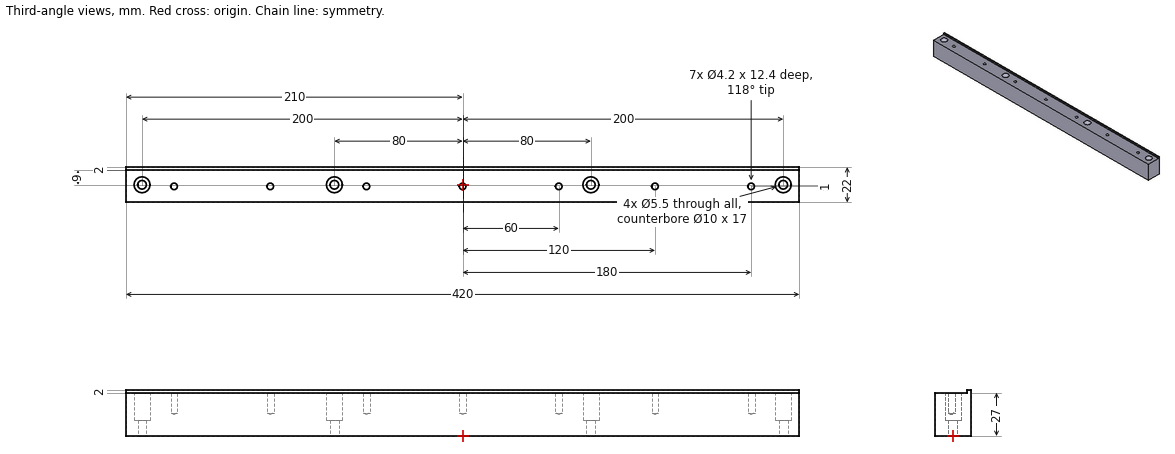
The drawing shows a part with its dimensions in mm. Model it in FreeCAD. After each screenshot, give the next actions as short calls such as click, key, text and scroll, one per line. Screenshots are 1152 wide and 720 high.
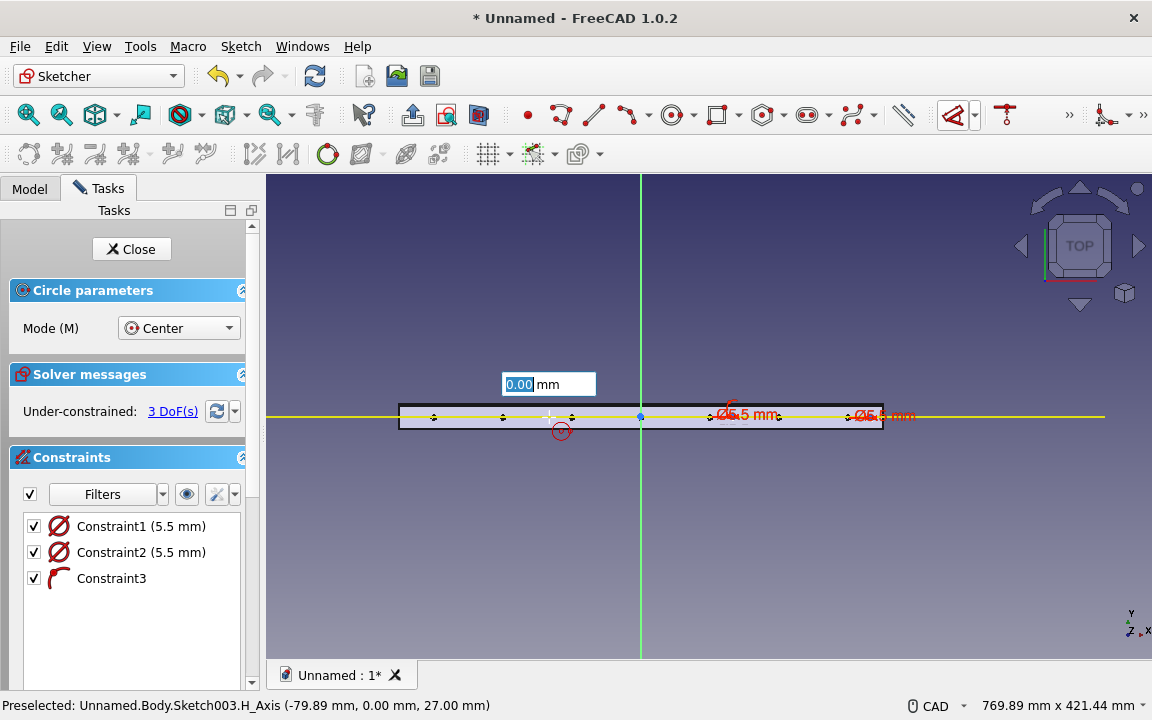
scroll(550, 414, up, 9)
move(548, 410)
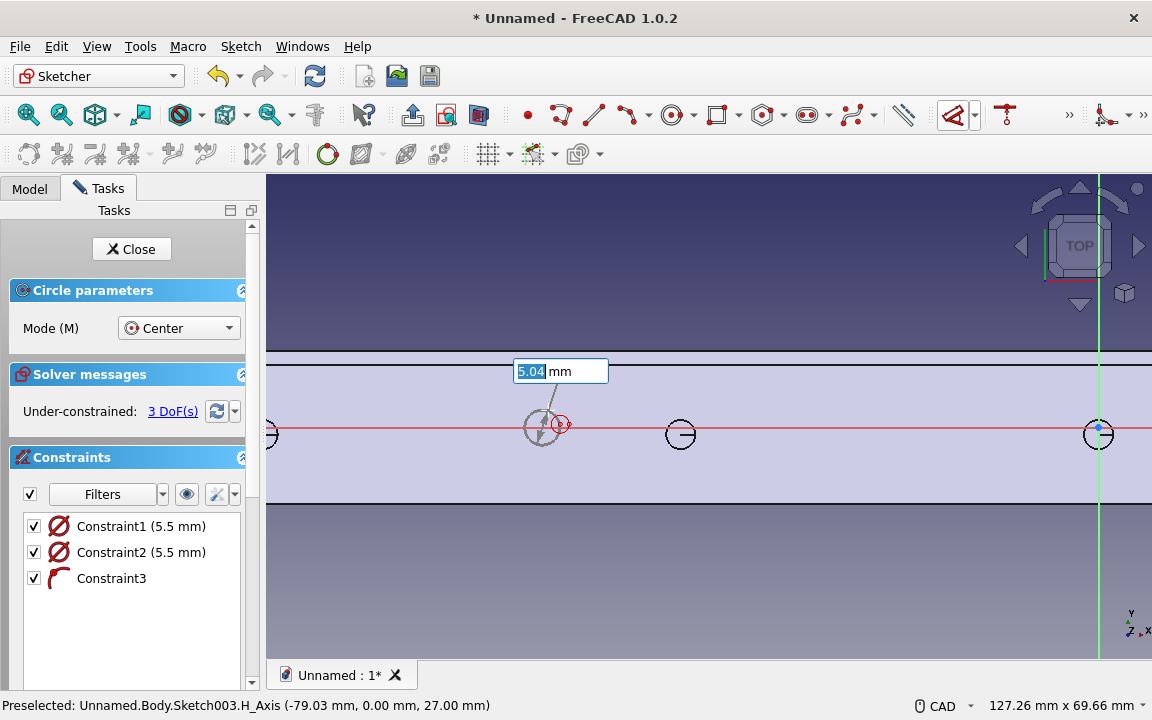
text(5.5)
key(Return)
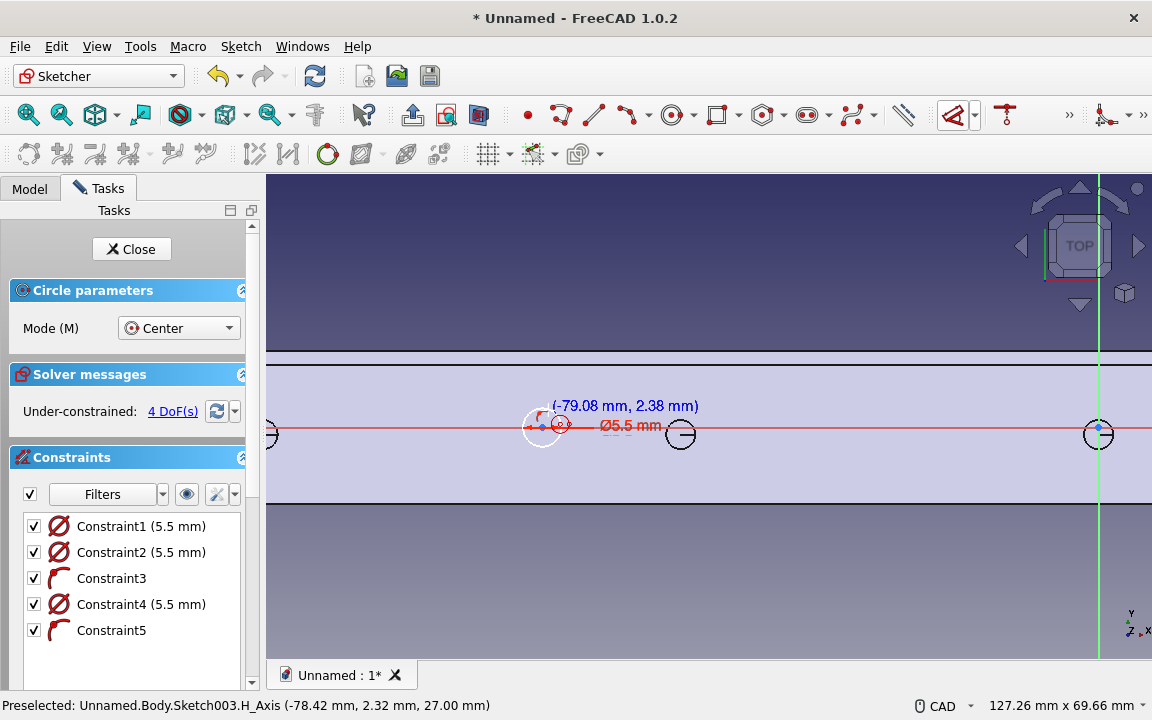
scroll(550, 414, down, 9)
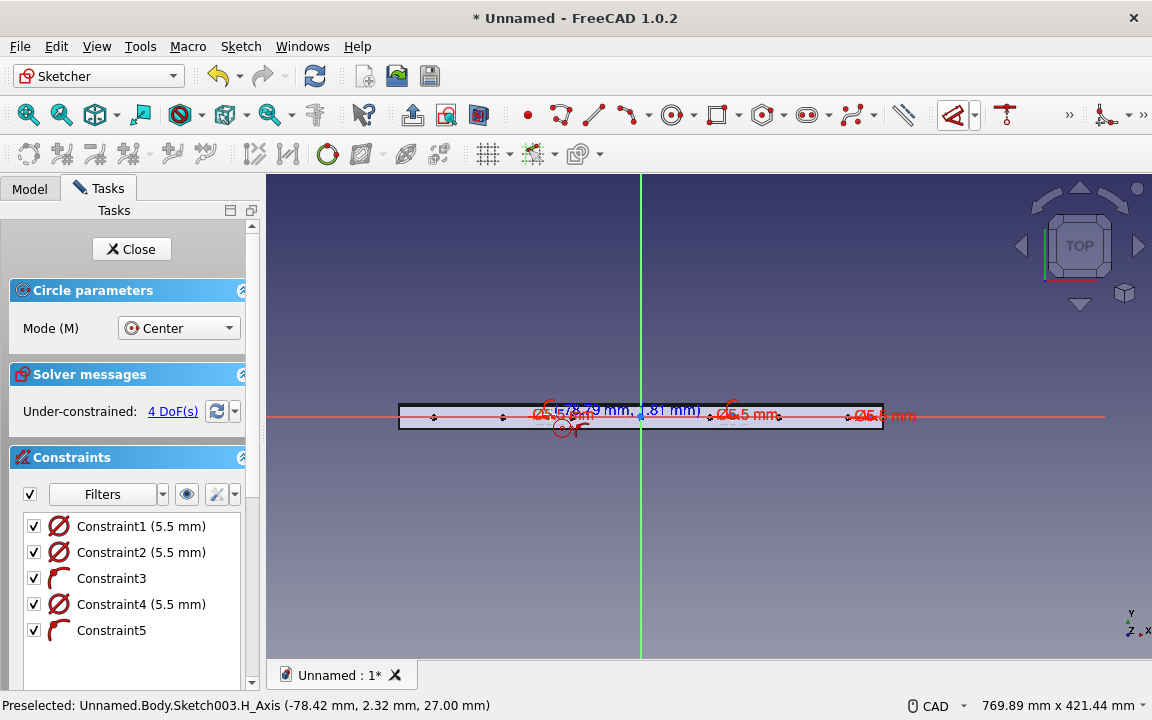
scroll(411, 417, up, 10)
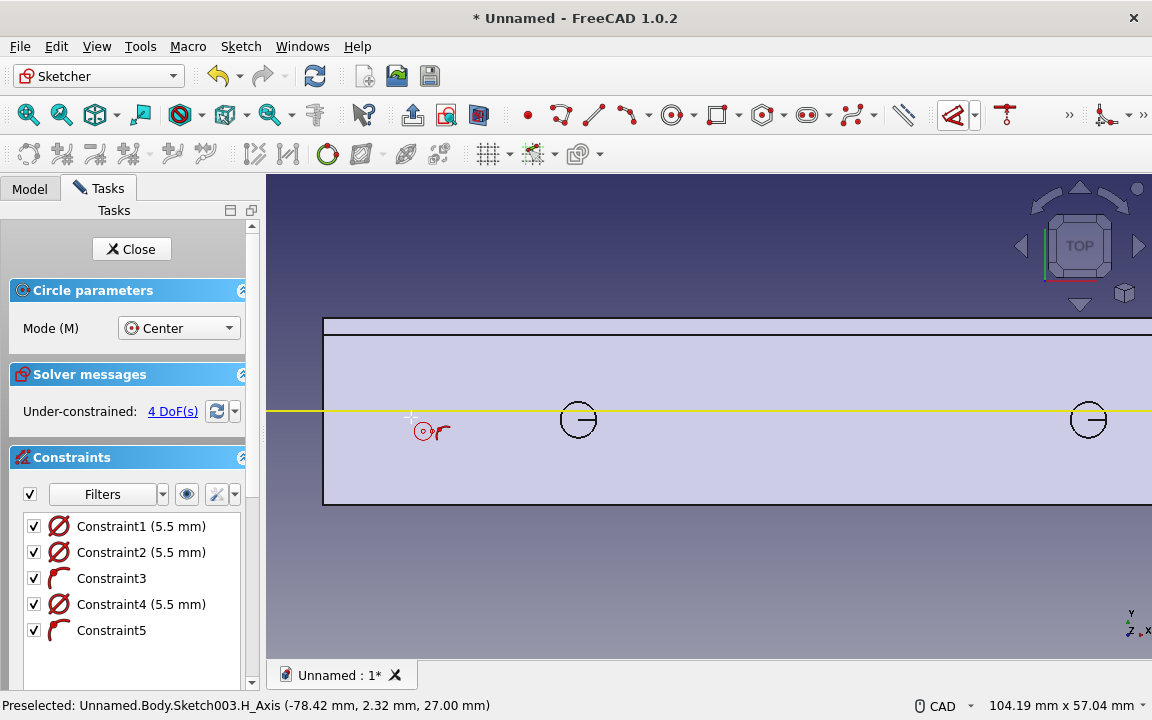
scroll(411, 417, down, 10)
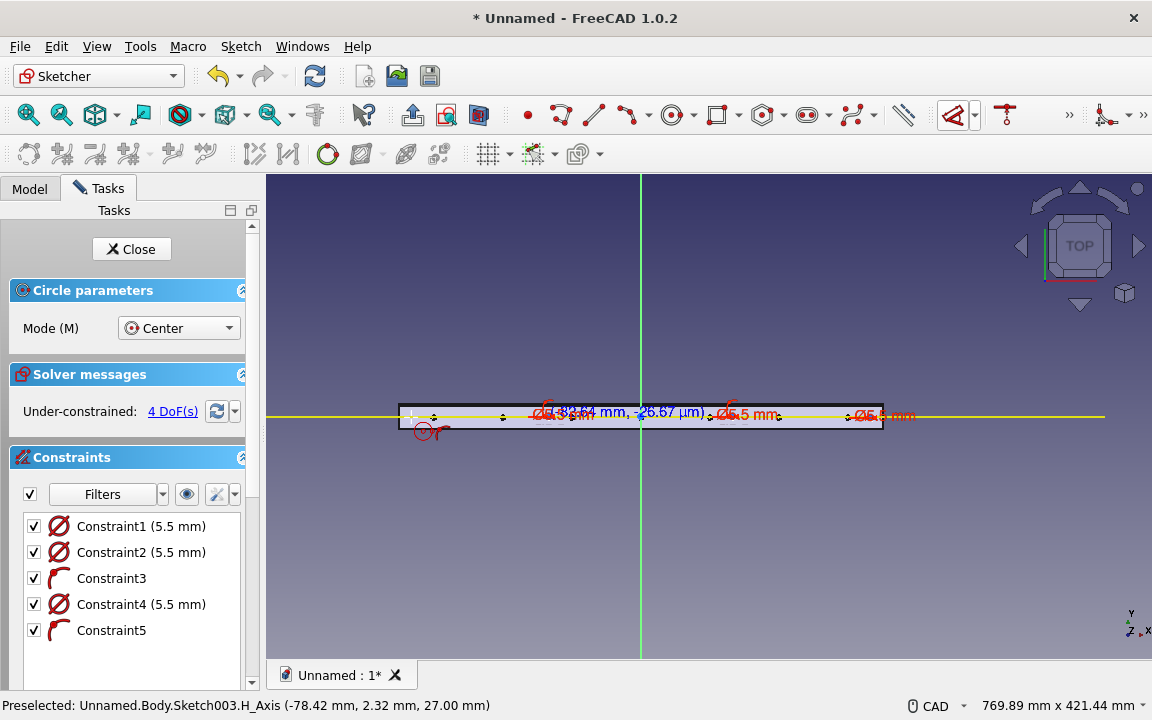
click(411, 417)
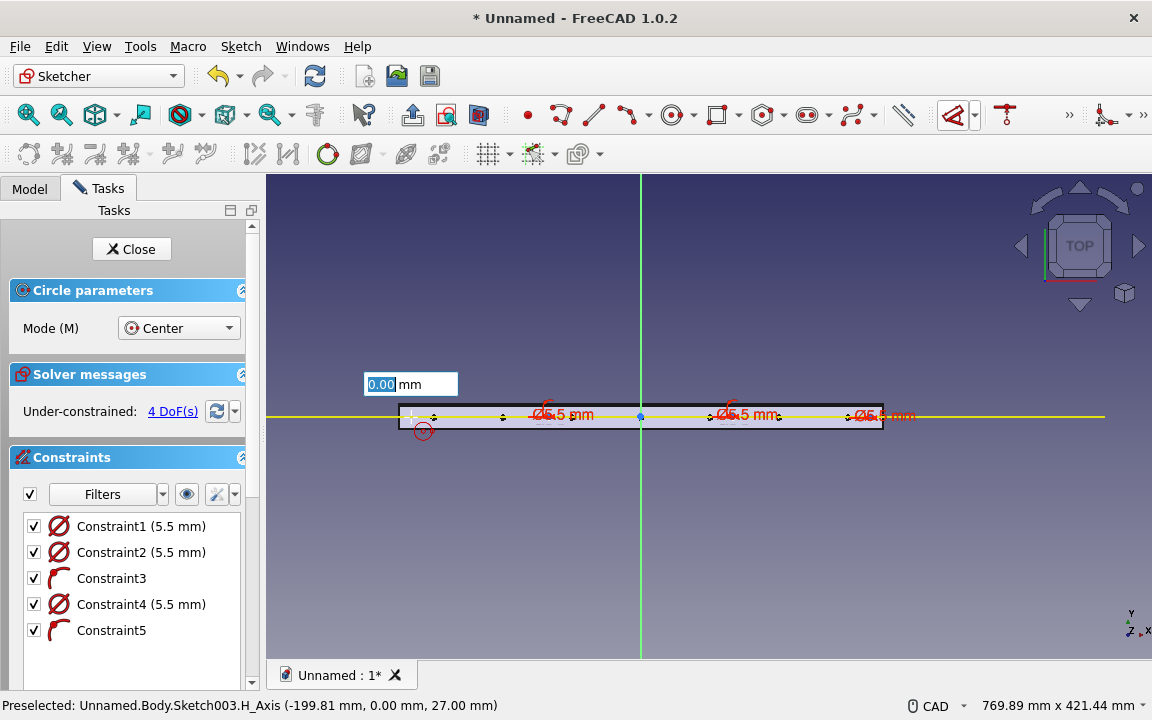
scroll(412, 414, up, 9)
move(410, 410)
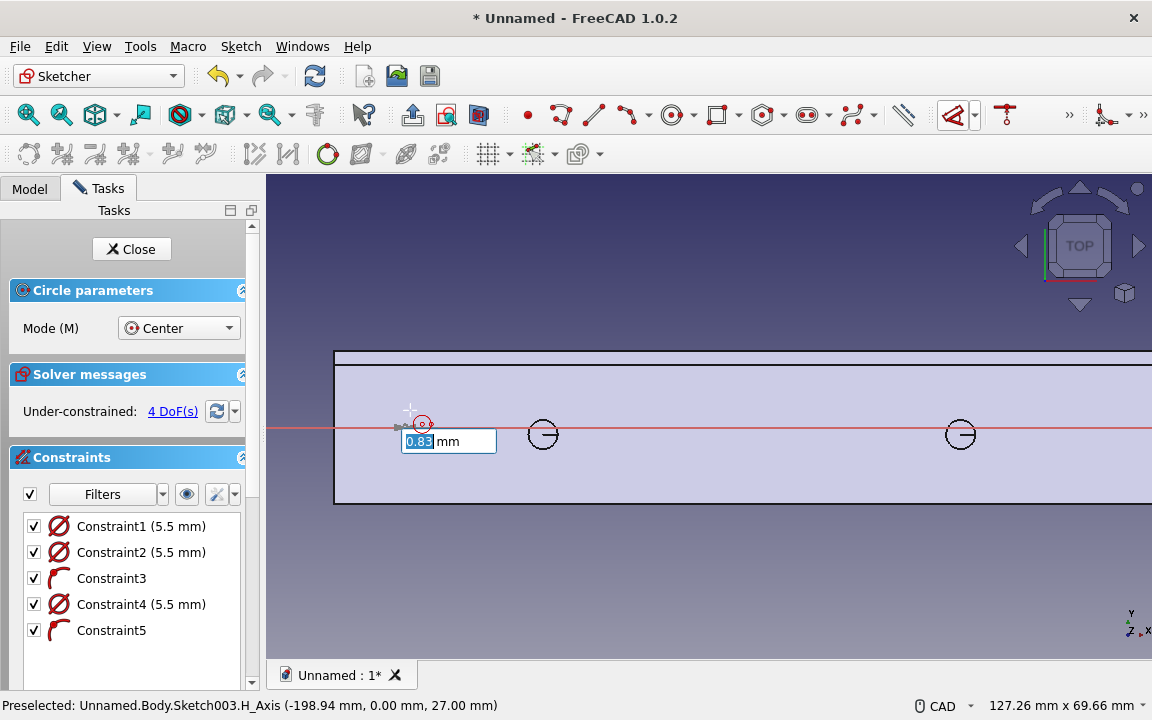
text(5.5)
key(Return)
key(Escape)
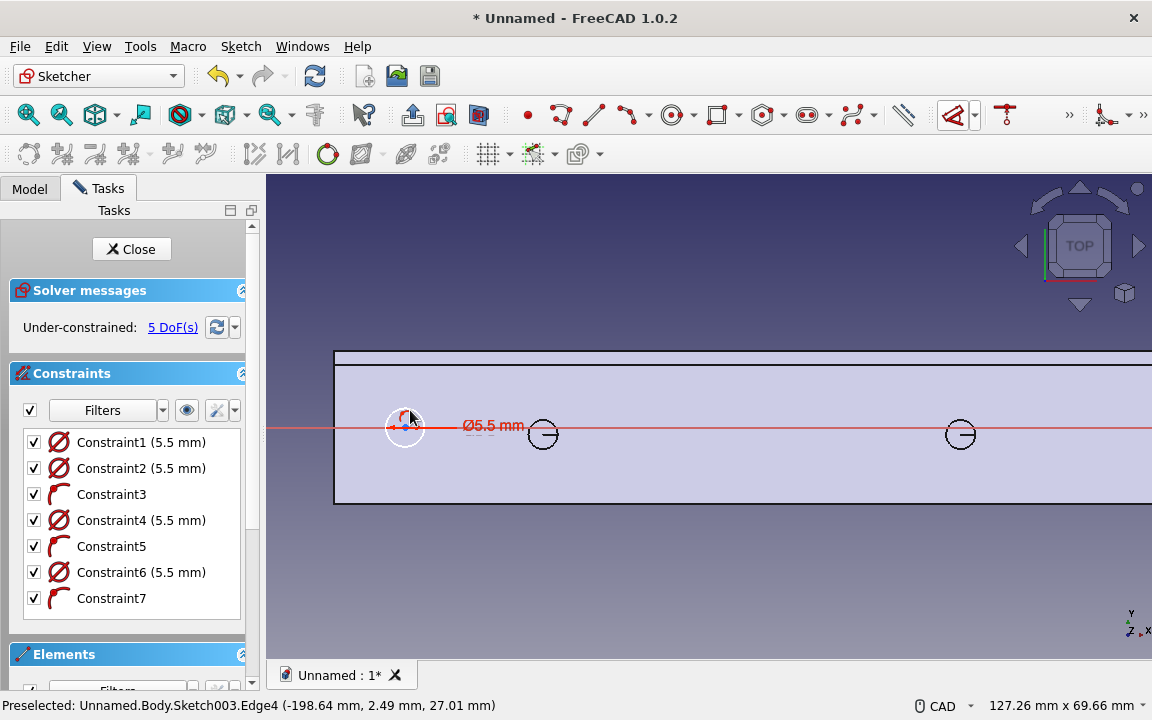
scroll(412, 414, down, 9)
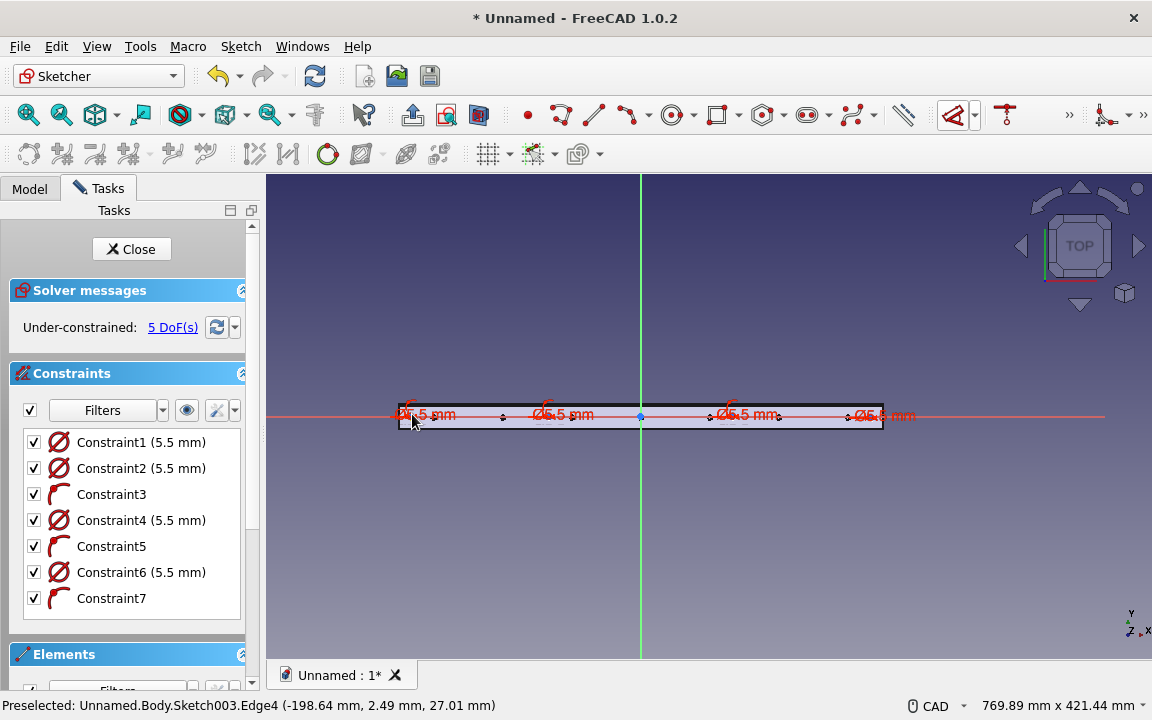
click(871, 418)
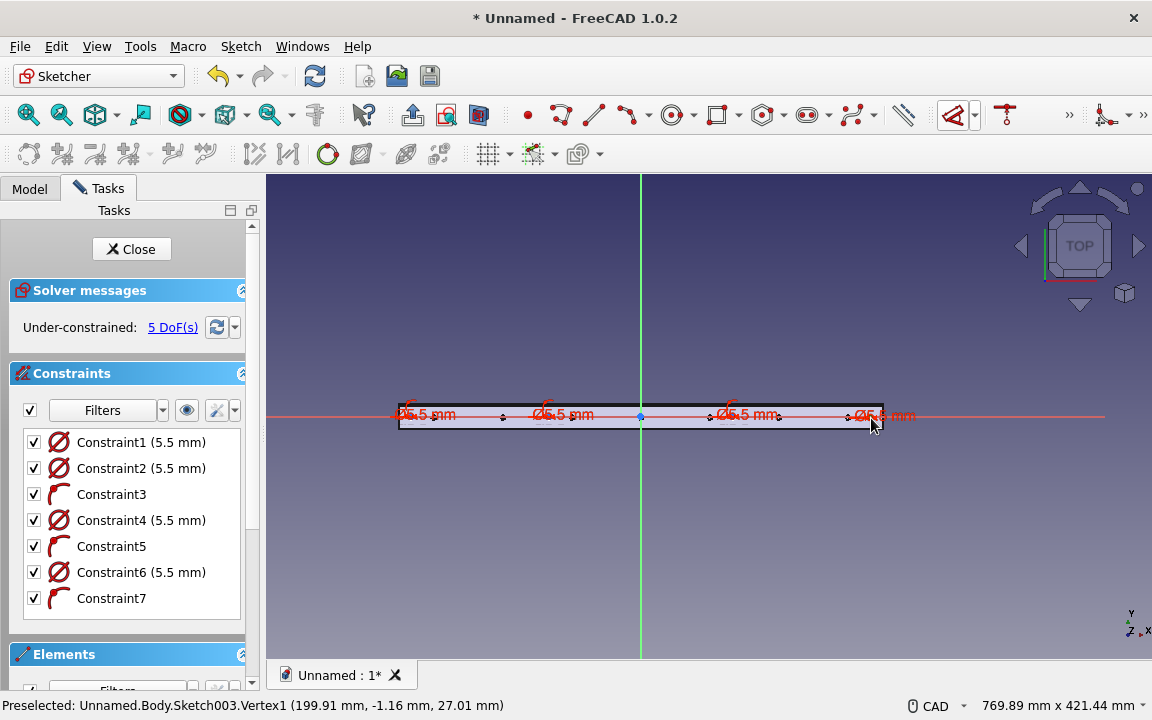
click(343, 417)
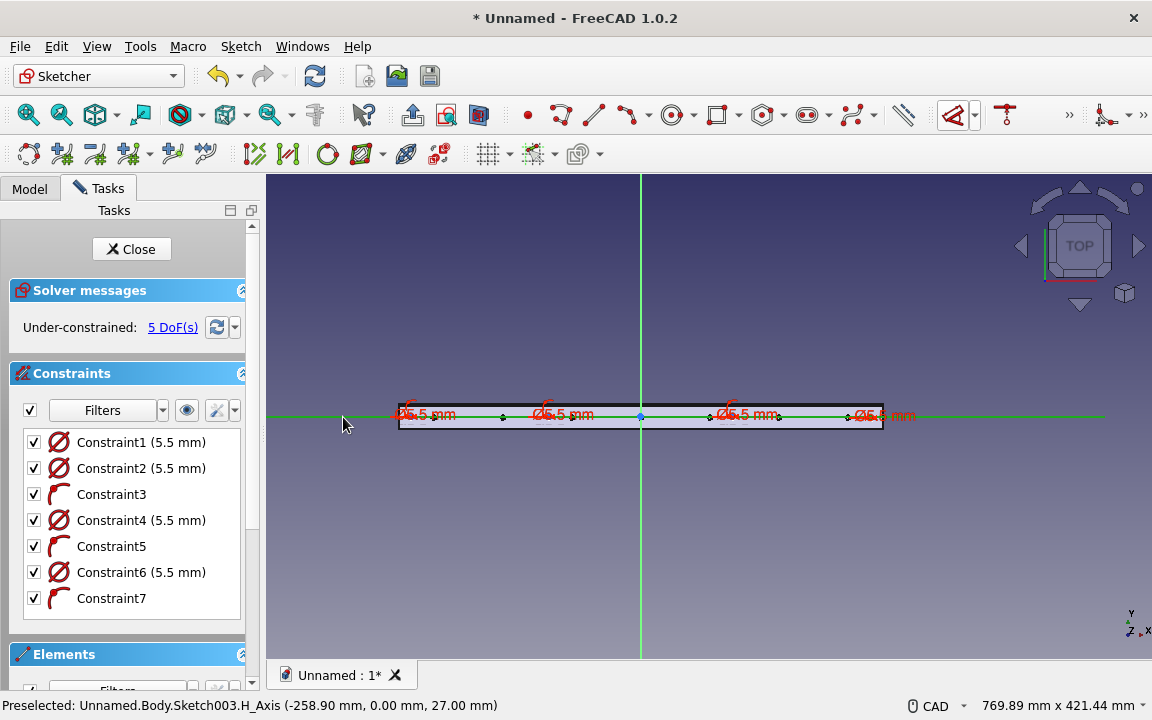
click(1005, 116)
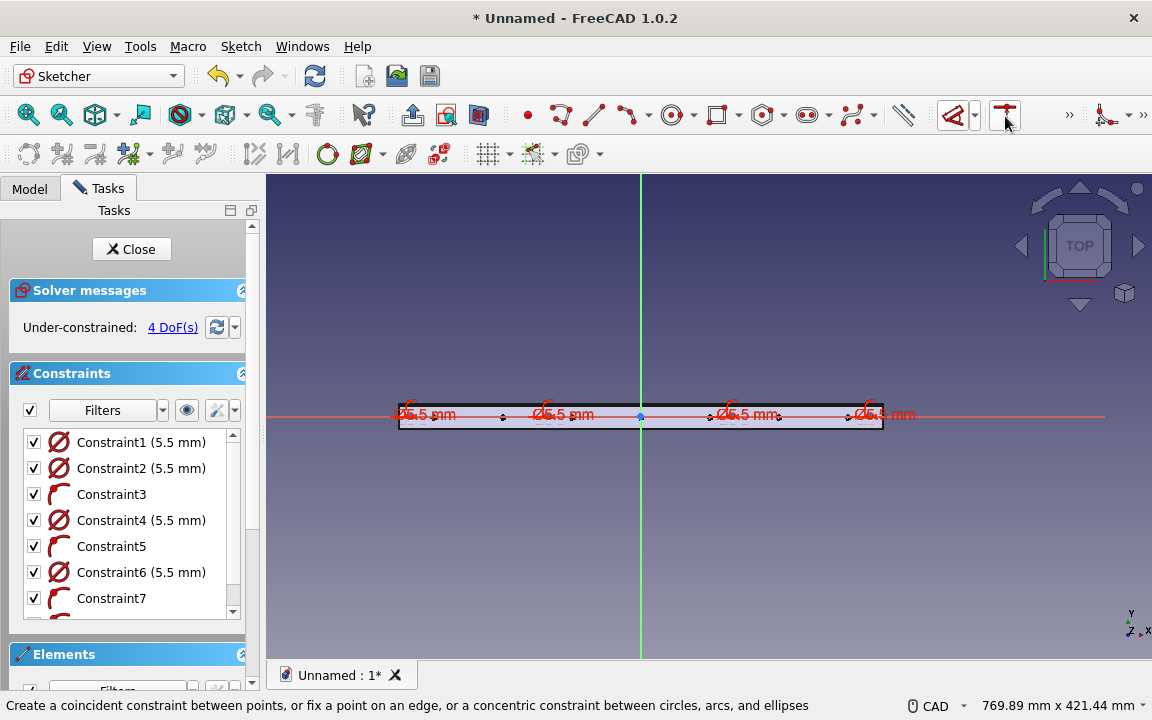
key(d)